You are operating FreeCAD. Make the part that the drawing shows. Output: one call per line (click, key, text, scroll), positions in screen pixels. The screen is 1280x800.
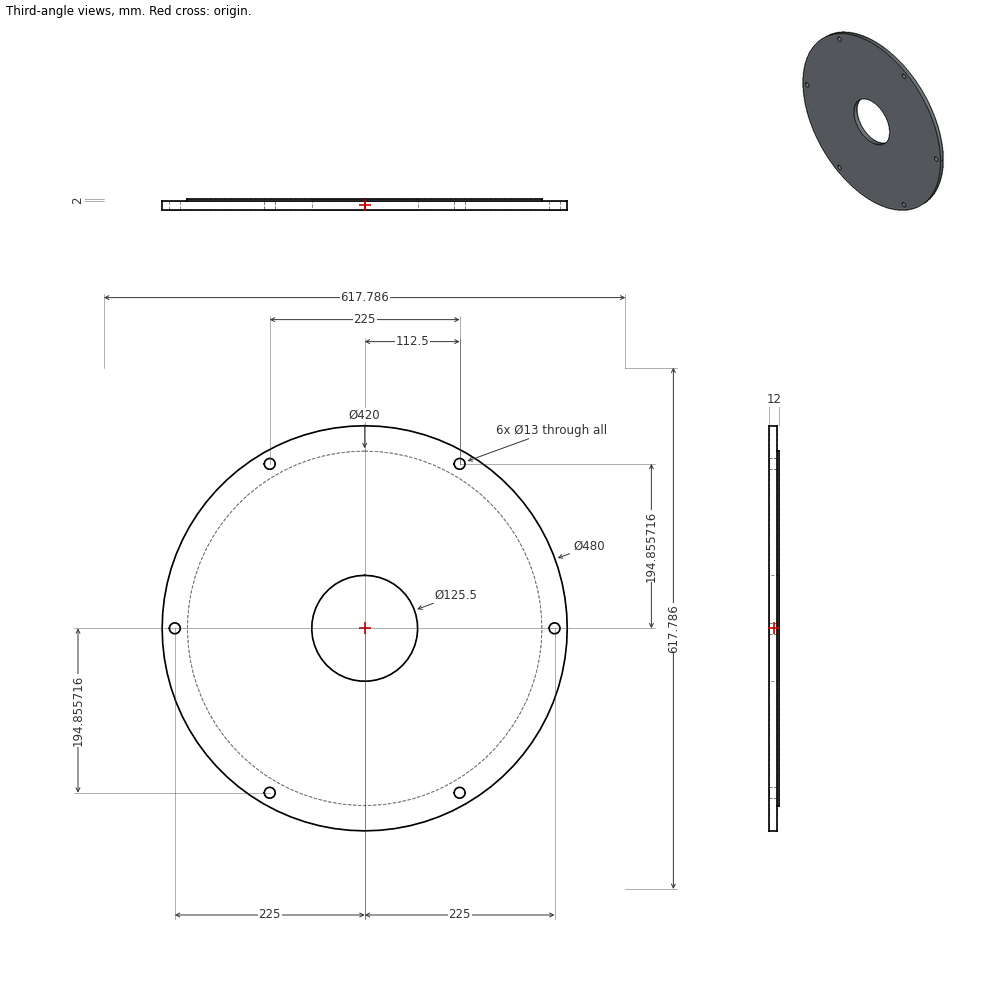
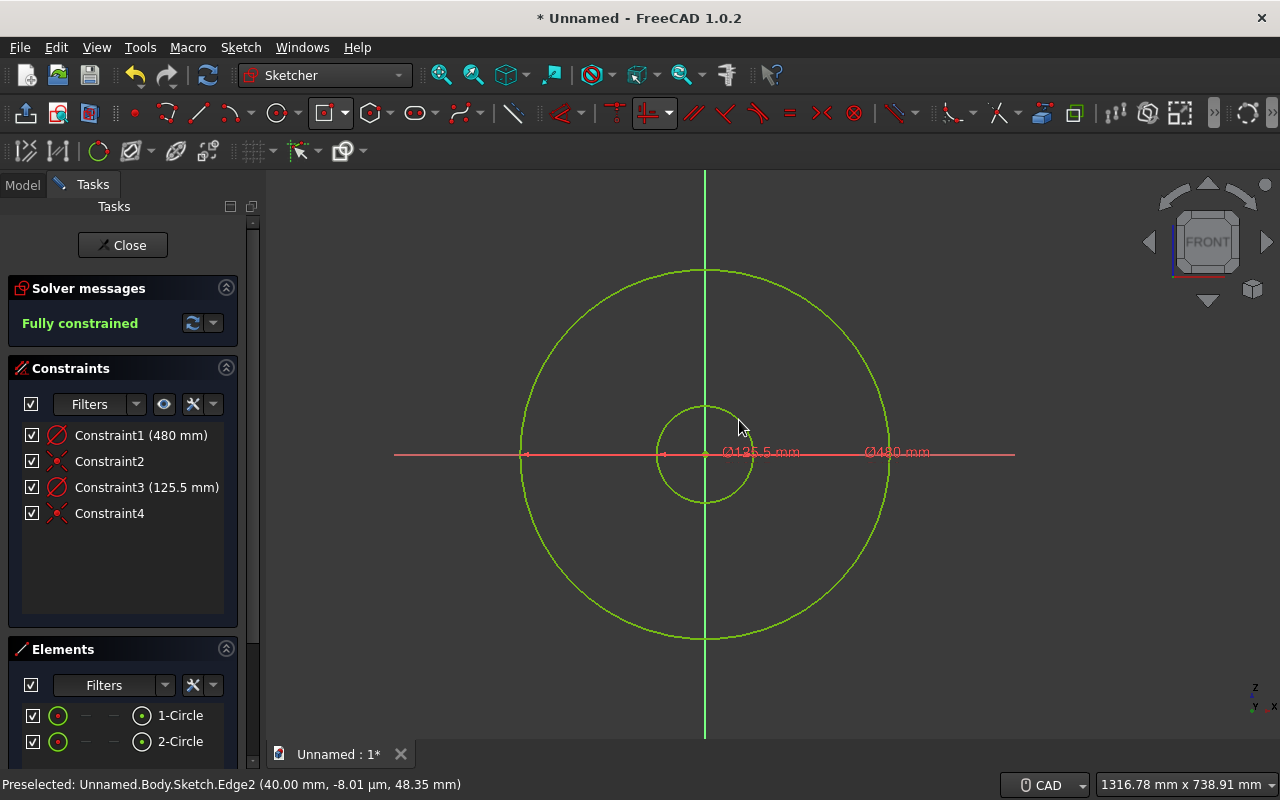
click(123, 245)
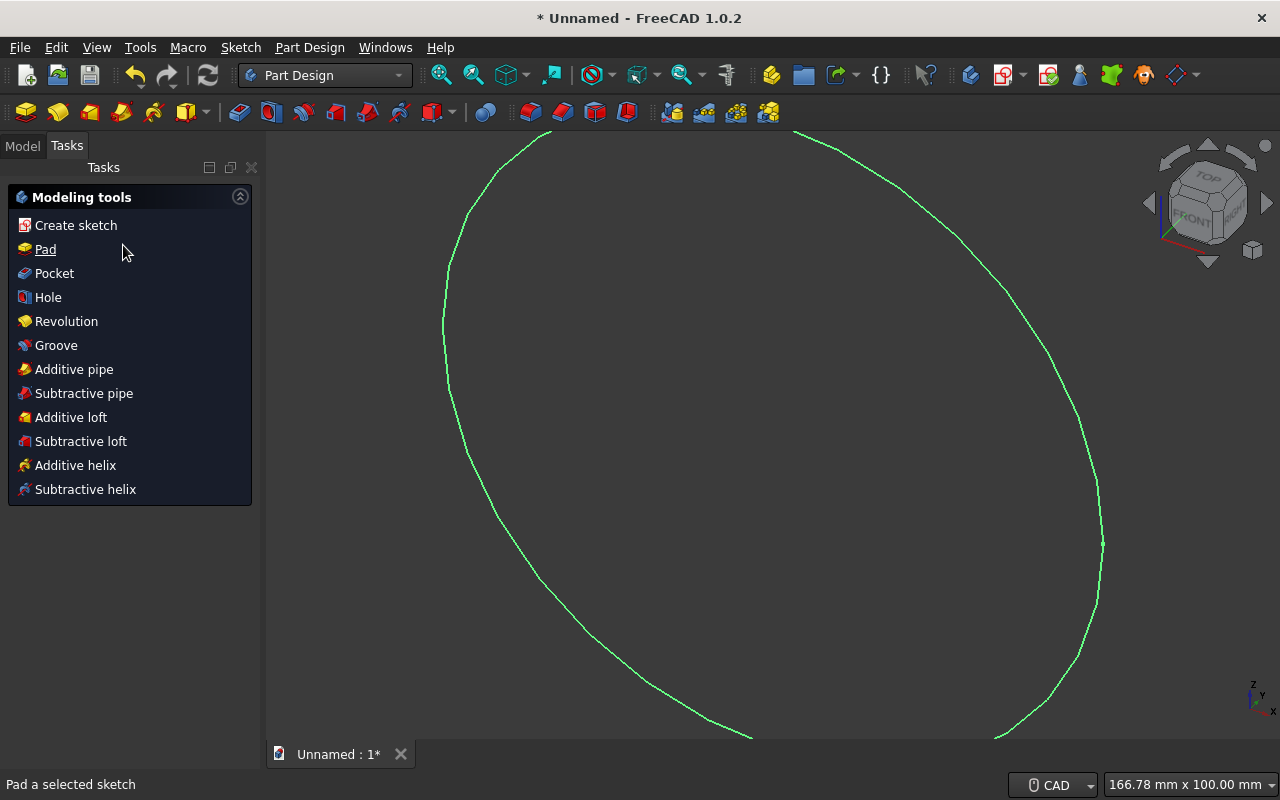
click(26, 112)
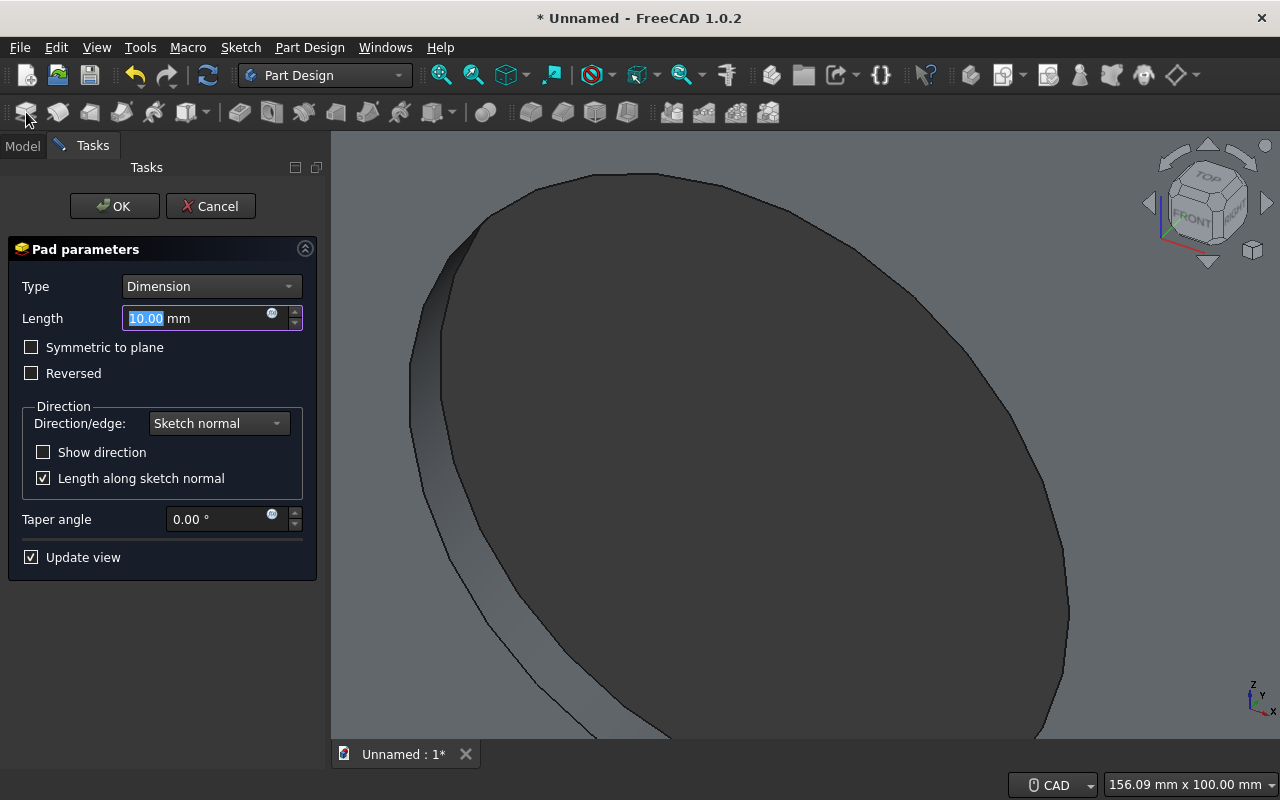
text(12)
key(Tab)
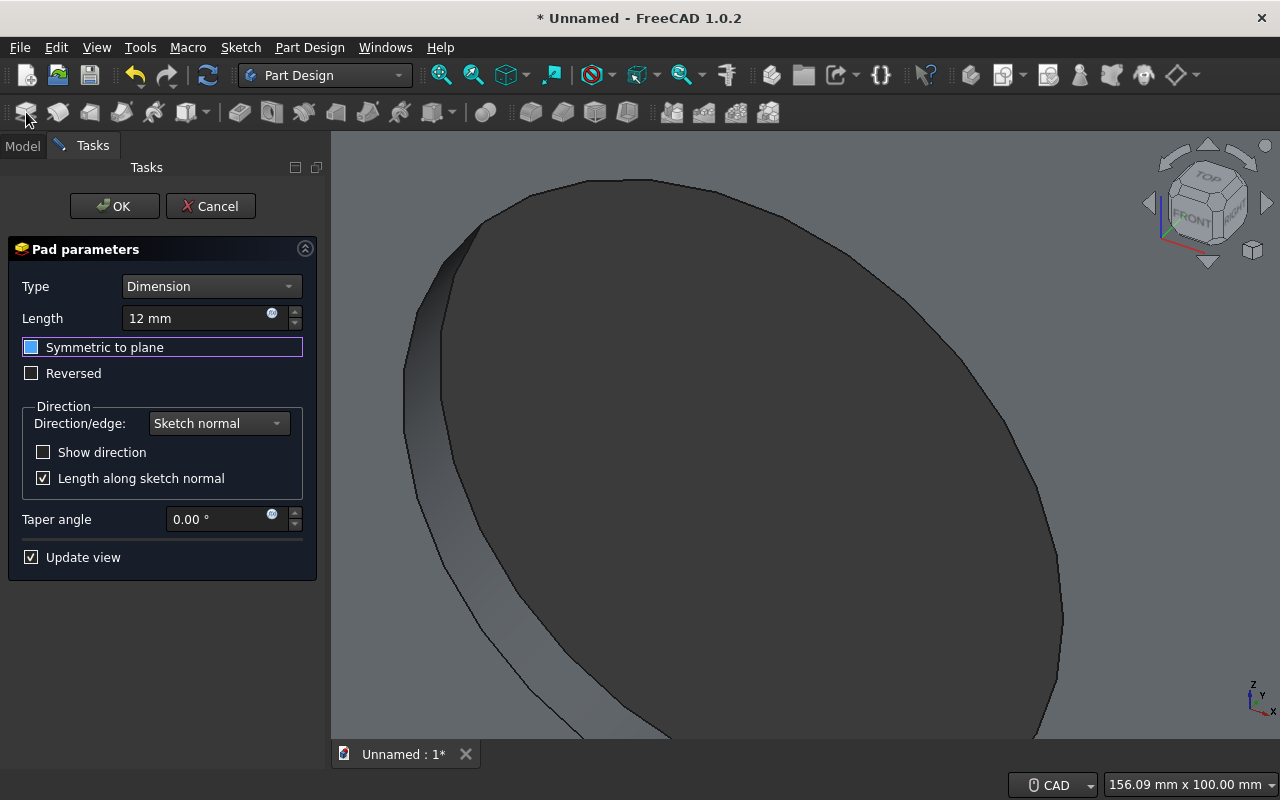
click(30, 347)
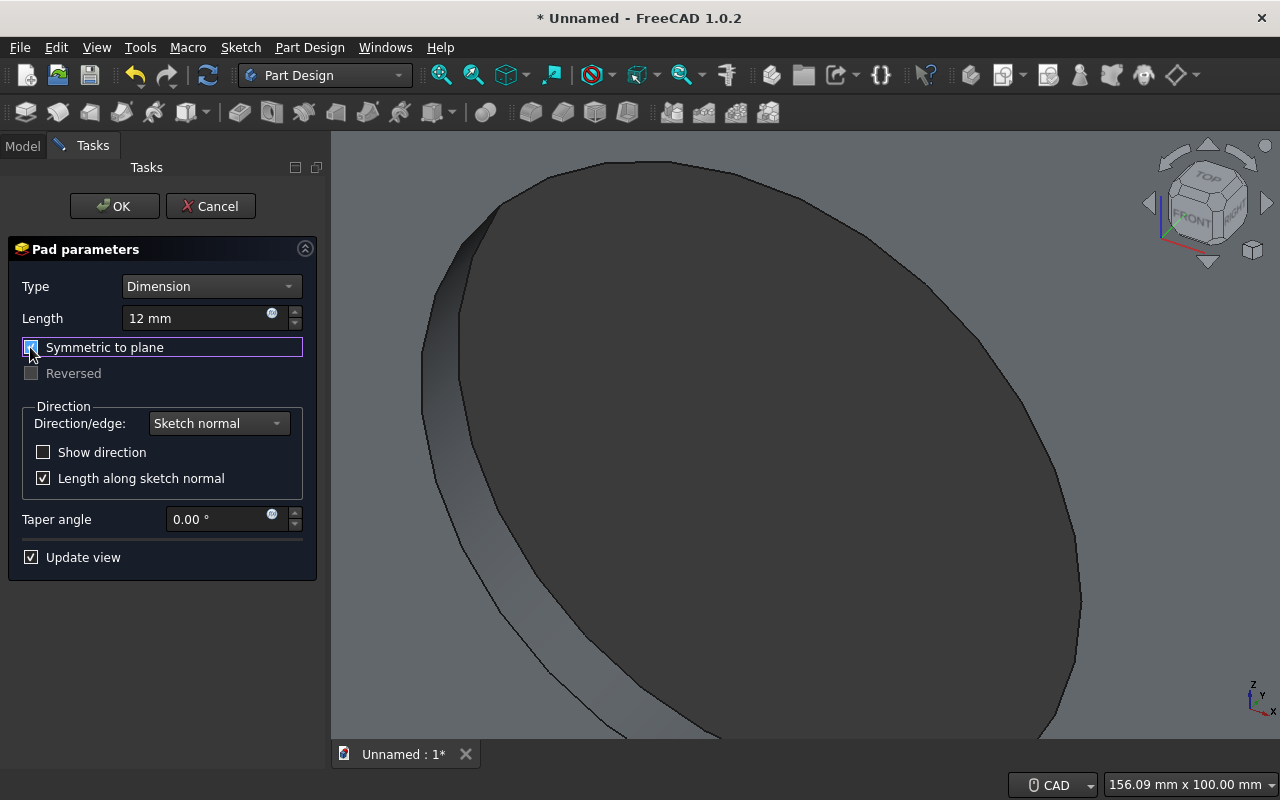
click(115, 206)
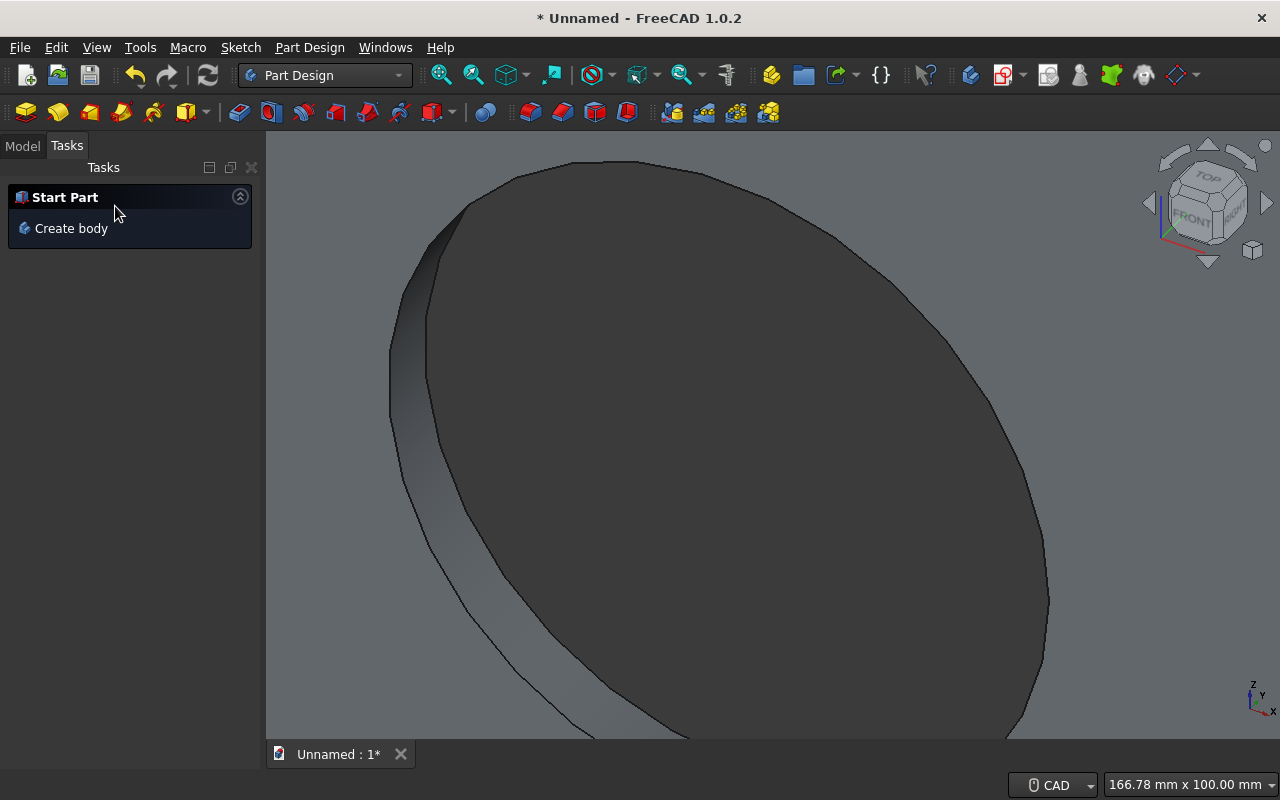
click(442, 76)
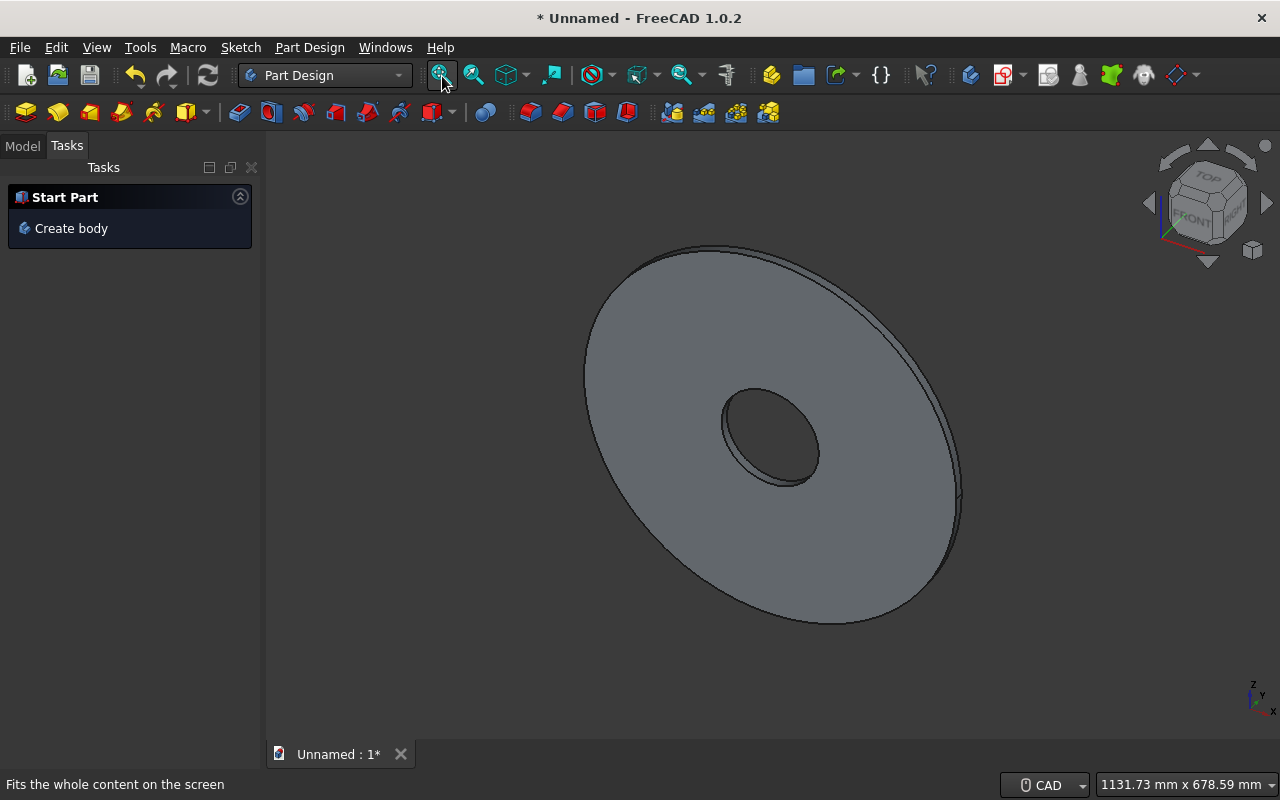
key(4)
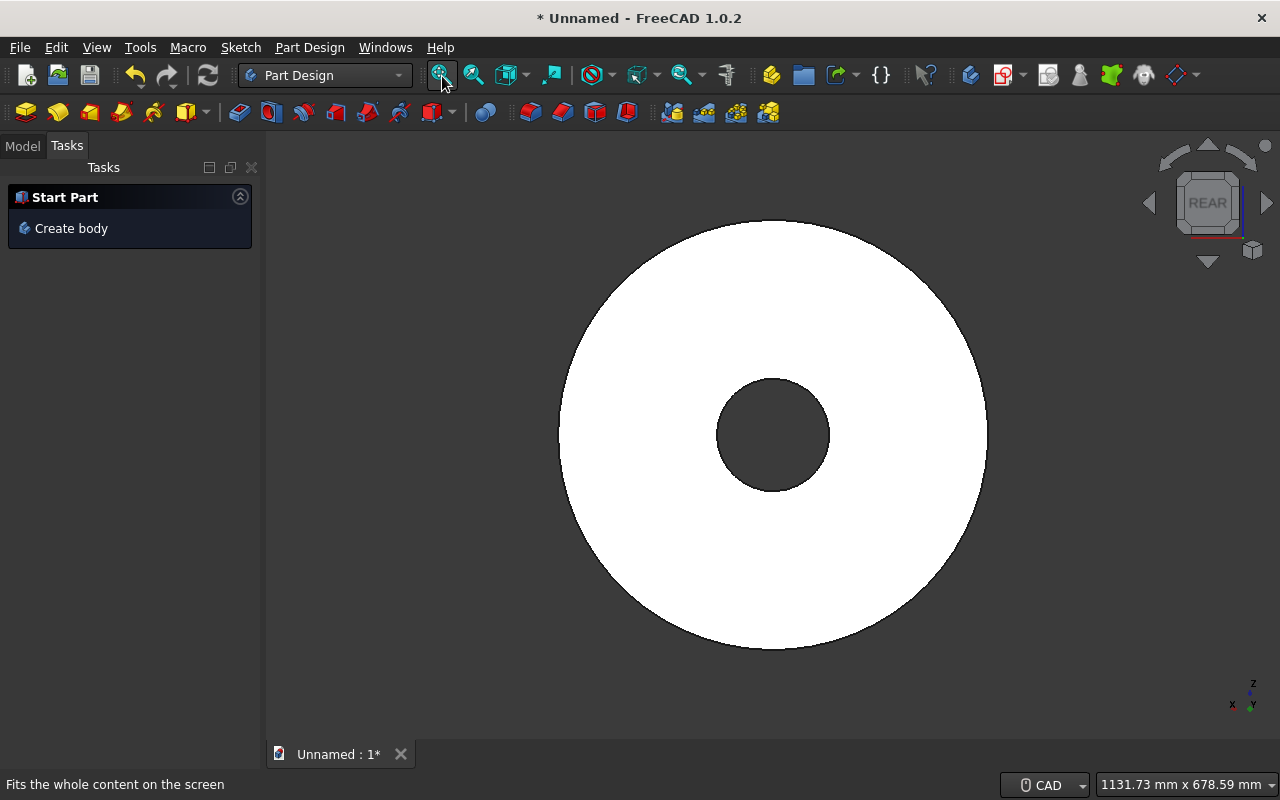
click(712, 557)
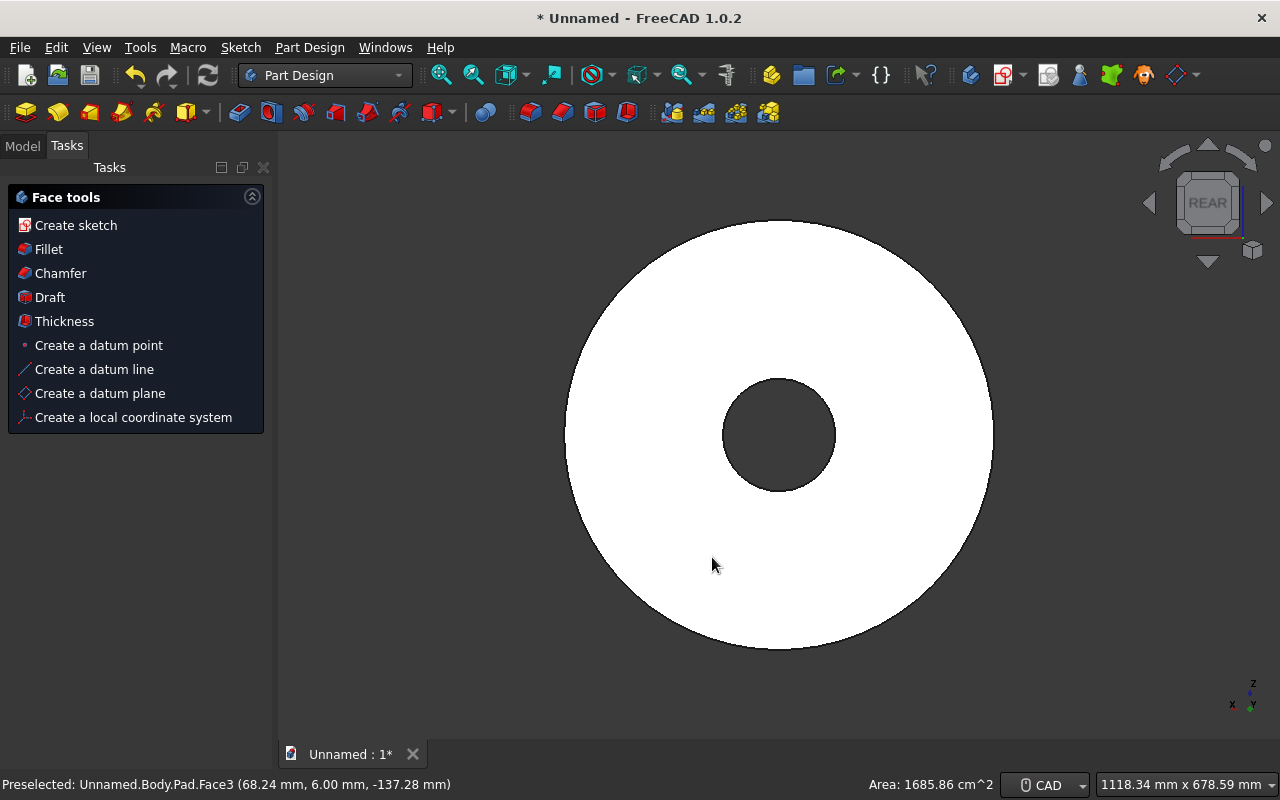
click(1004, 76)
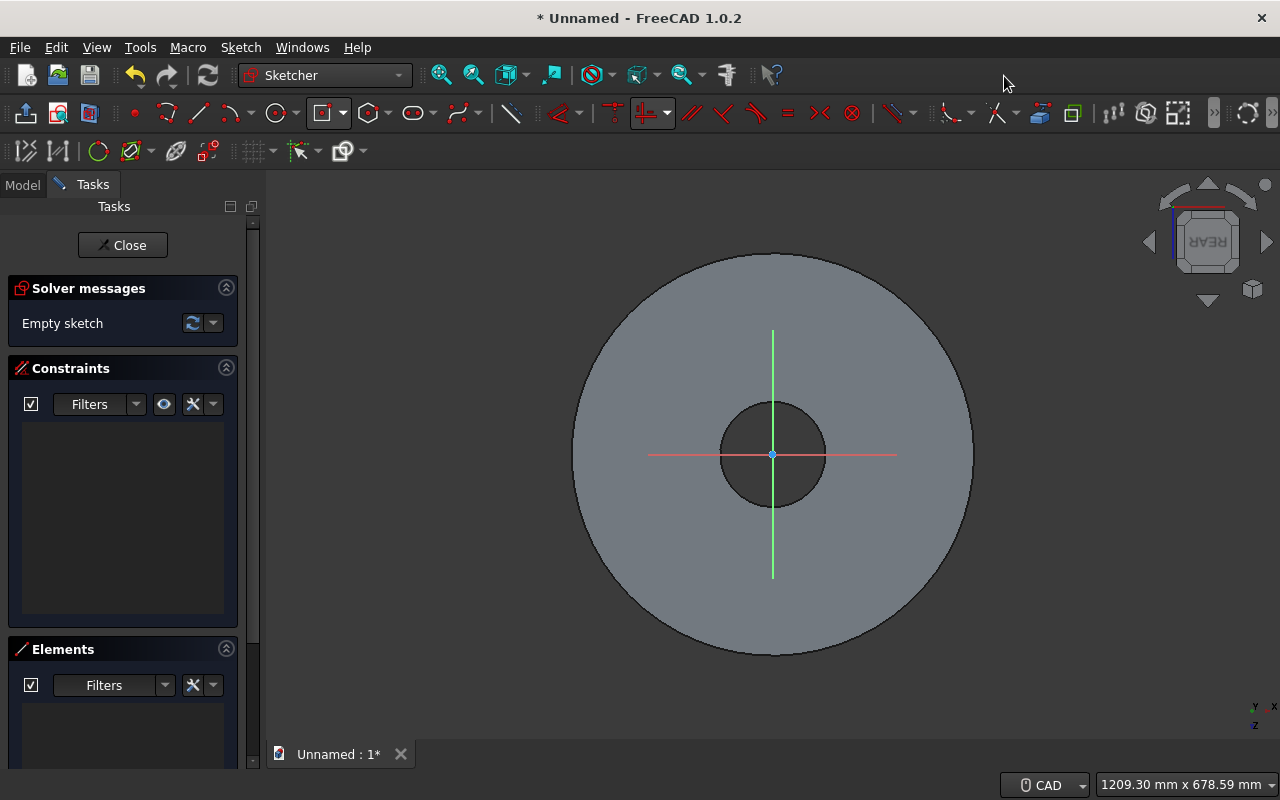
click(276, 114)